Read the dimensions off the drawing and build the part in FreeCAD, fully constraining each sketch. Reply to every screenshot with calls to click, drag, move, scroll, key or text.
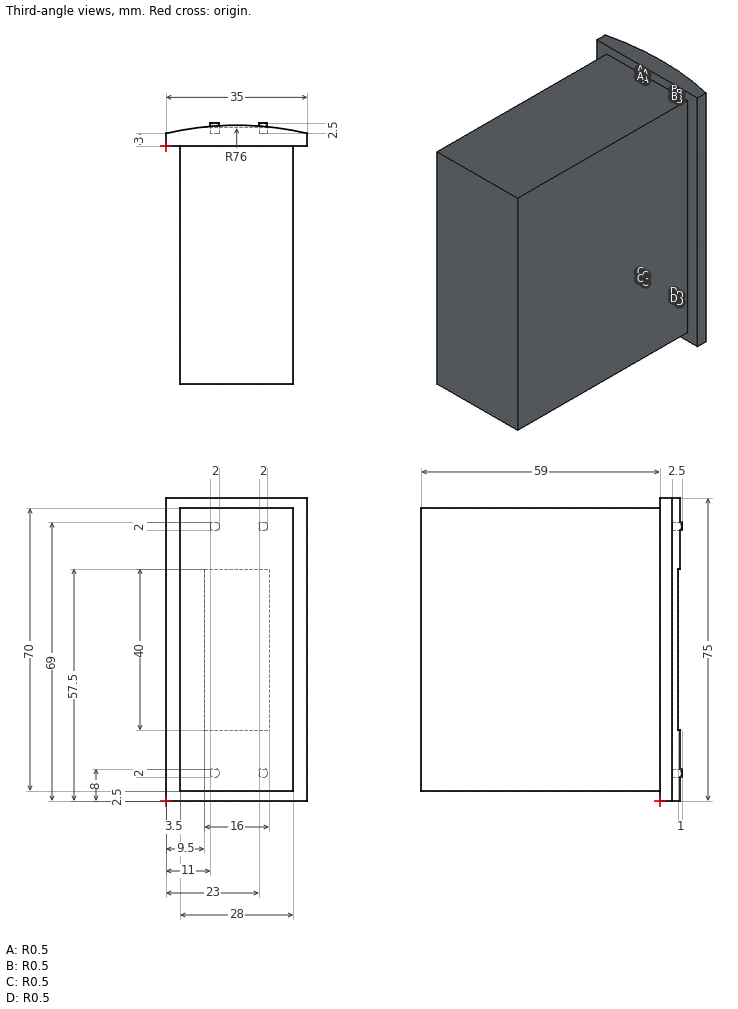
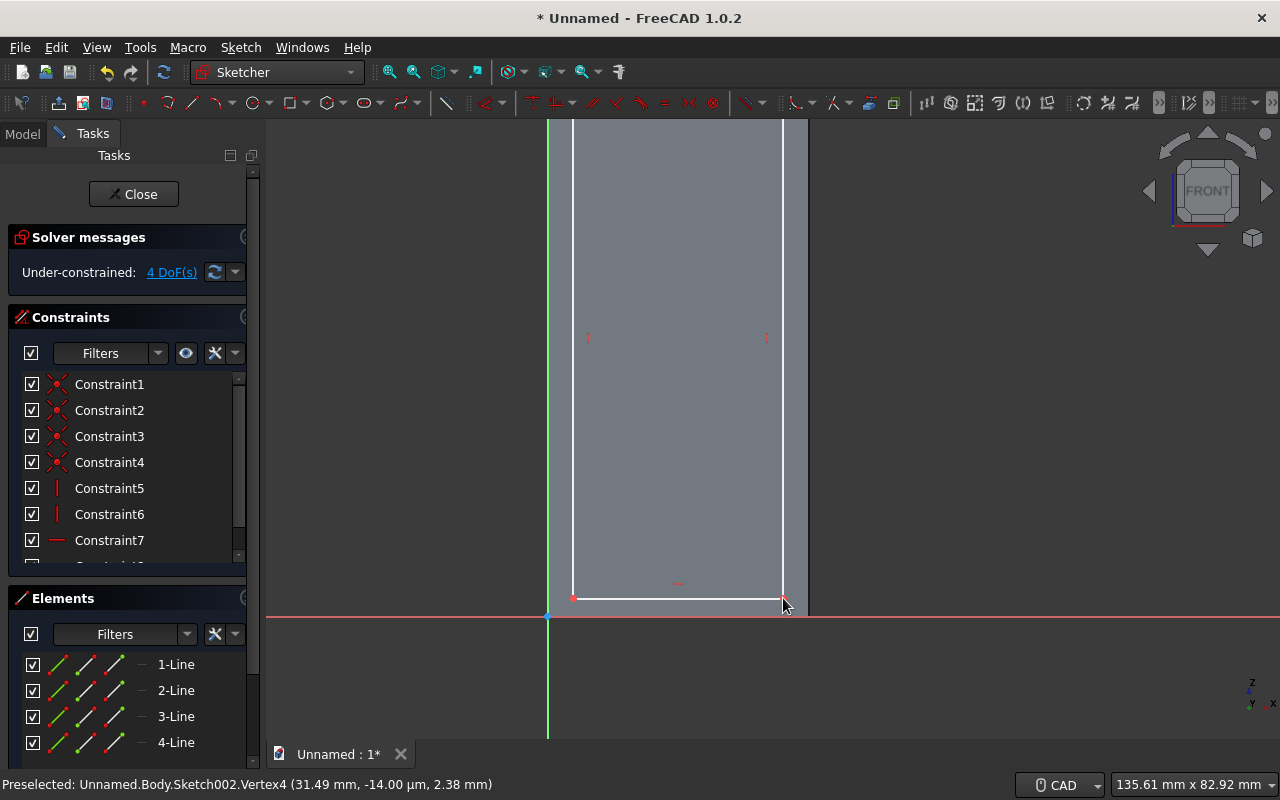
key(d)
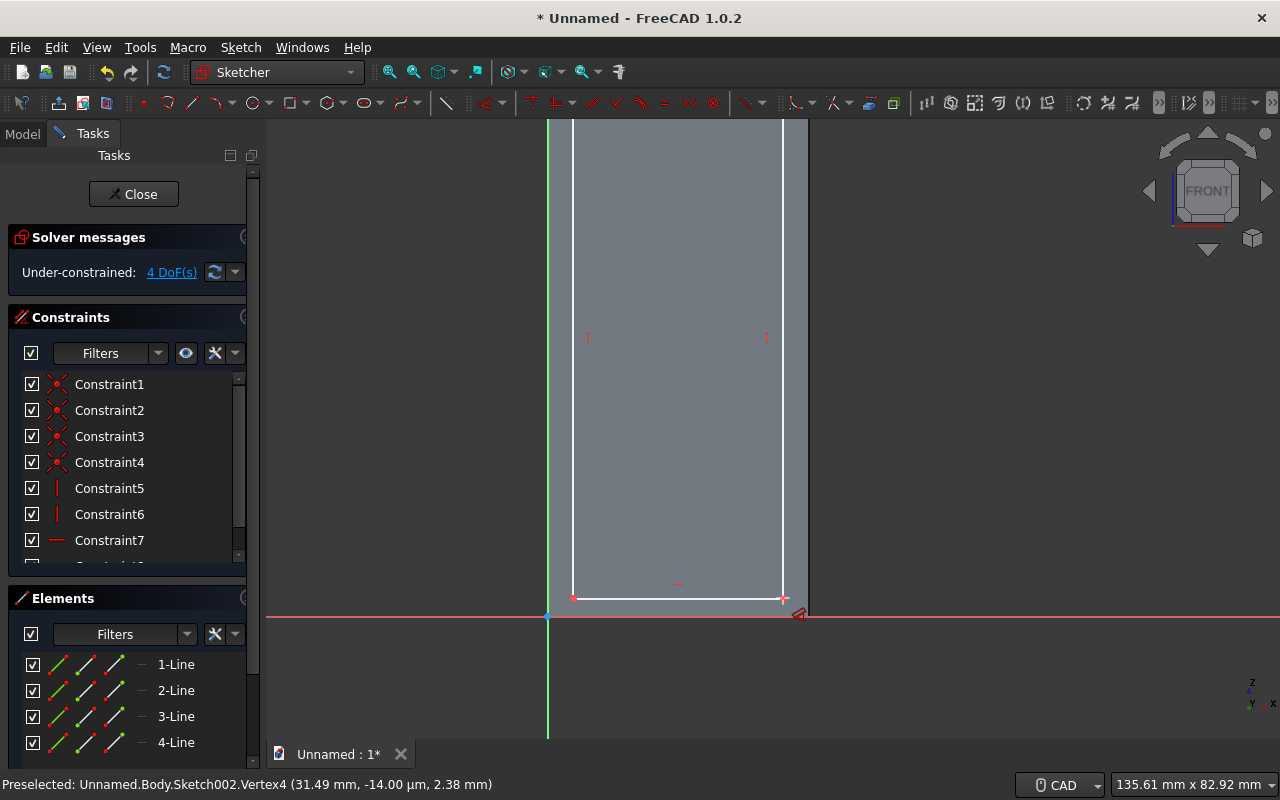
click(573, 233)
click(607, 373)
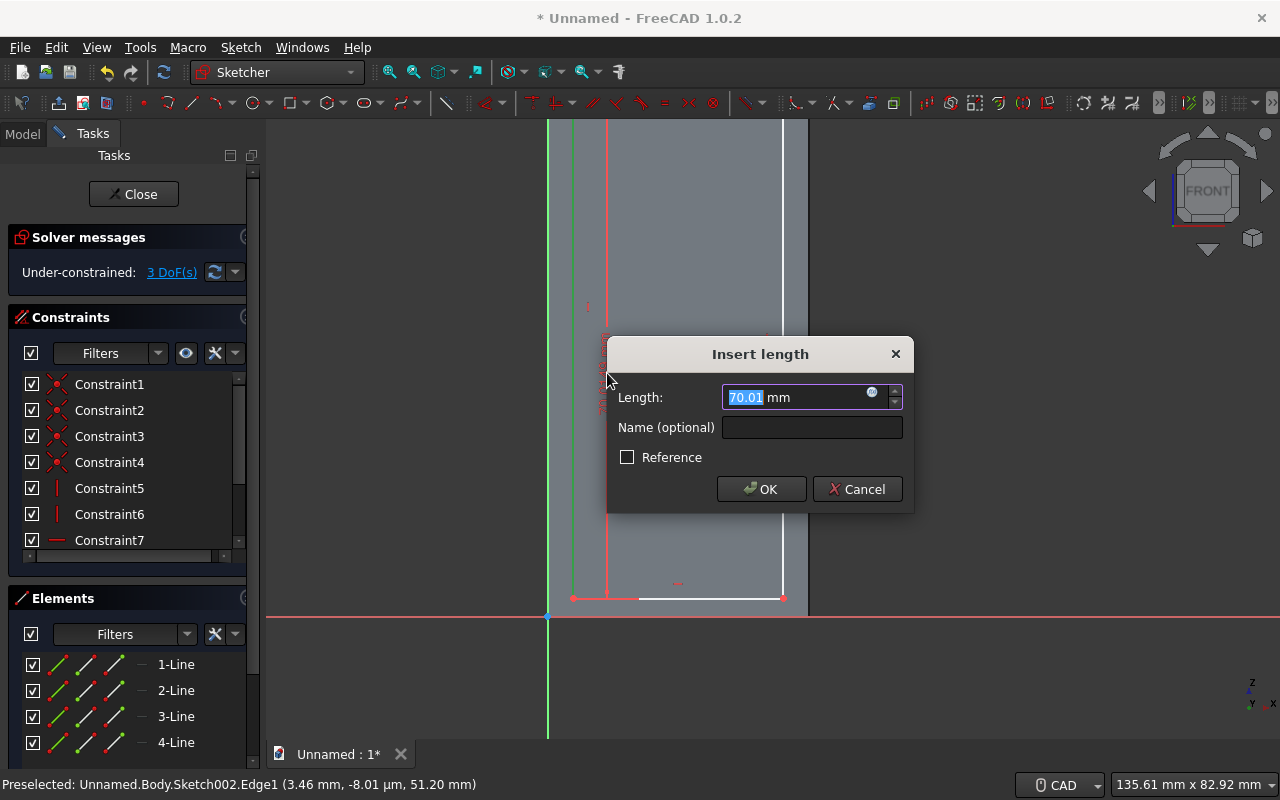
text(70)
key(Return)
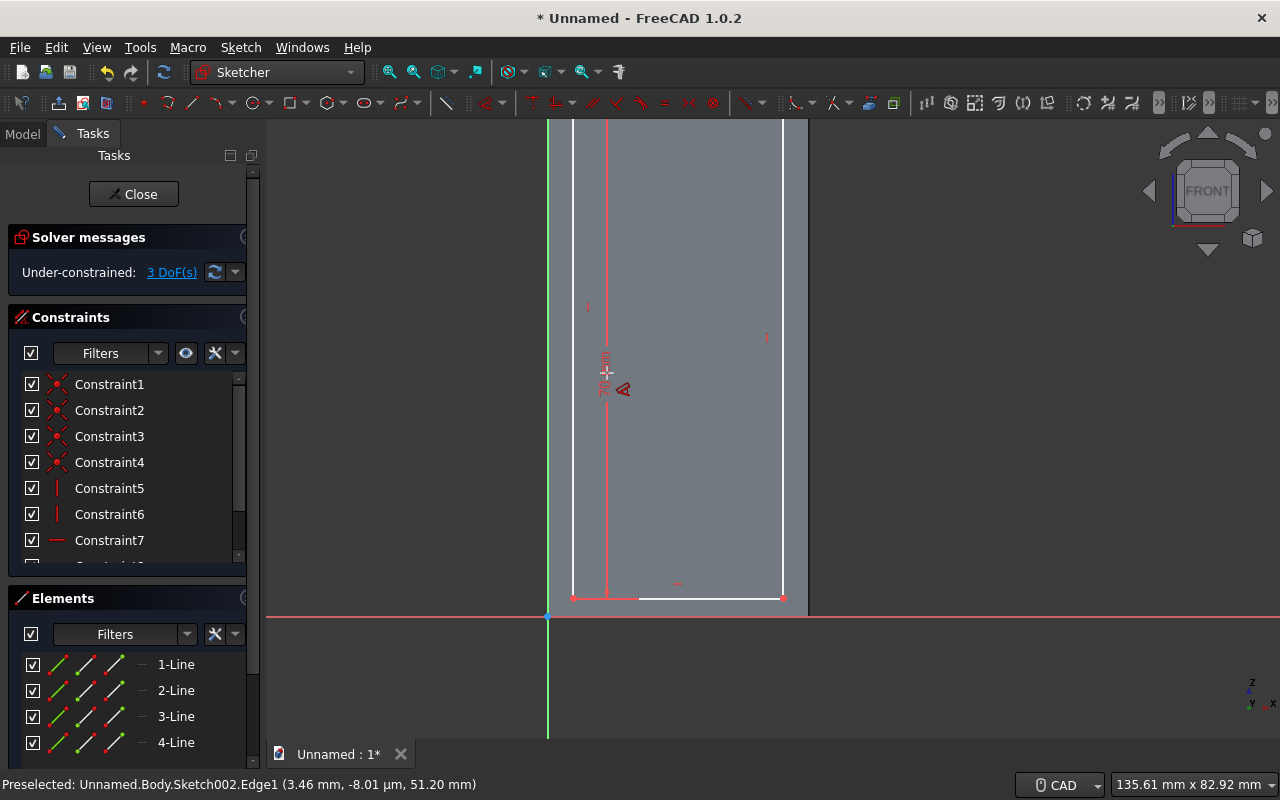
click(636, 599)
click(678, 633)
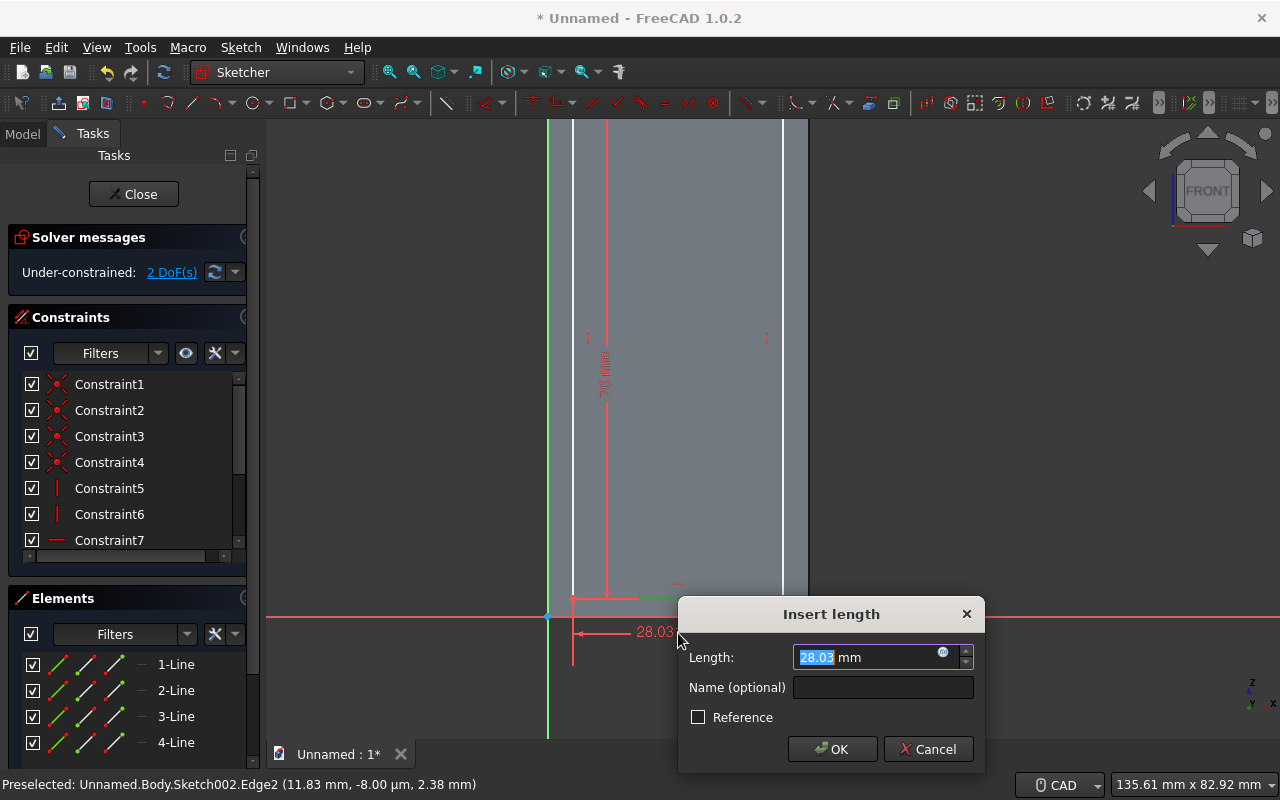
text(28)
key(Return)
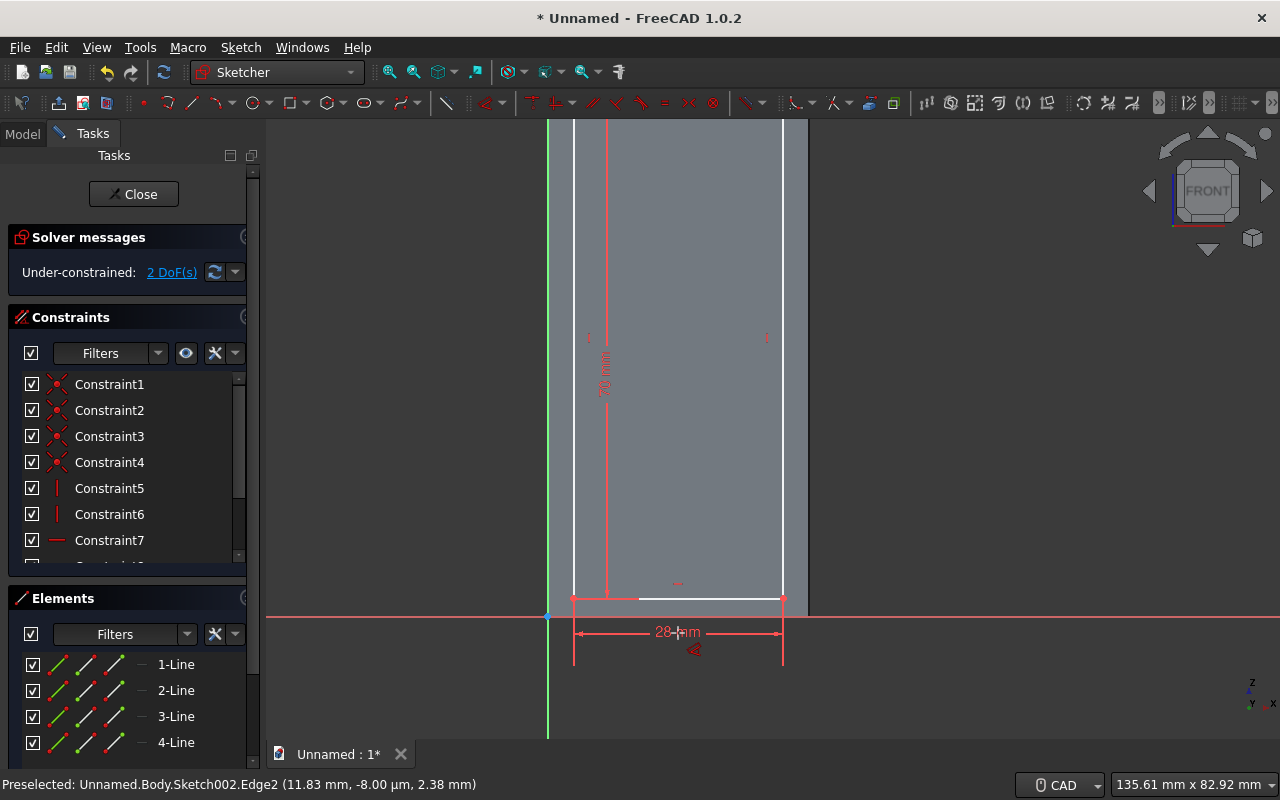
scroll(784, 598, down, 2)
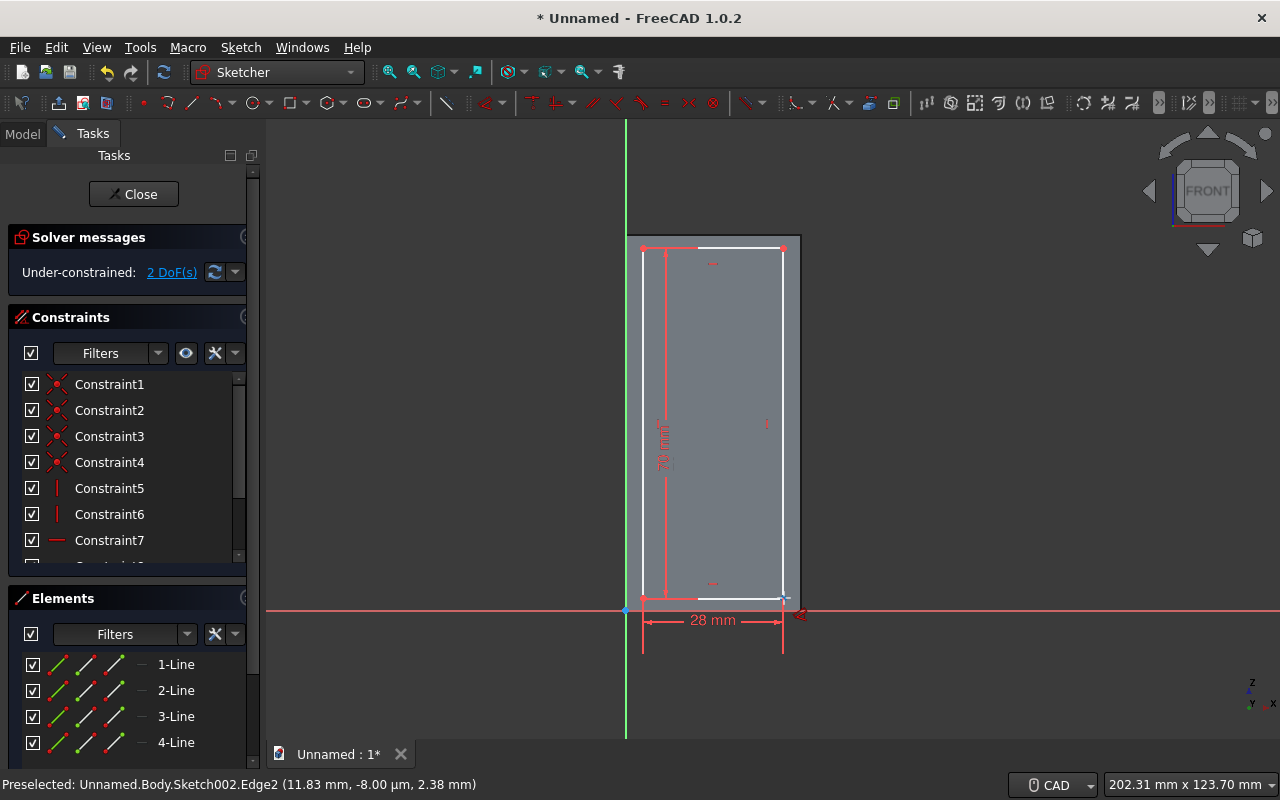
scroll(643, 248, up, 5)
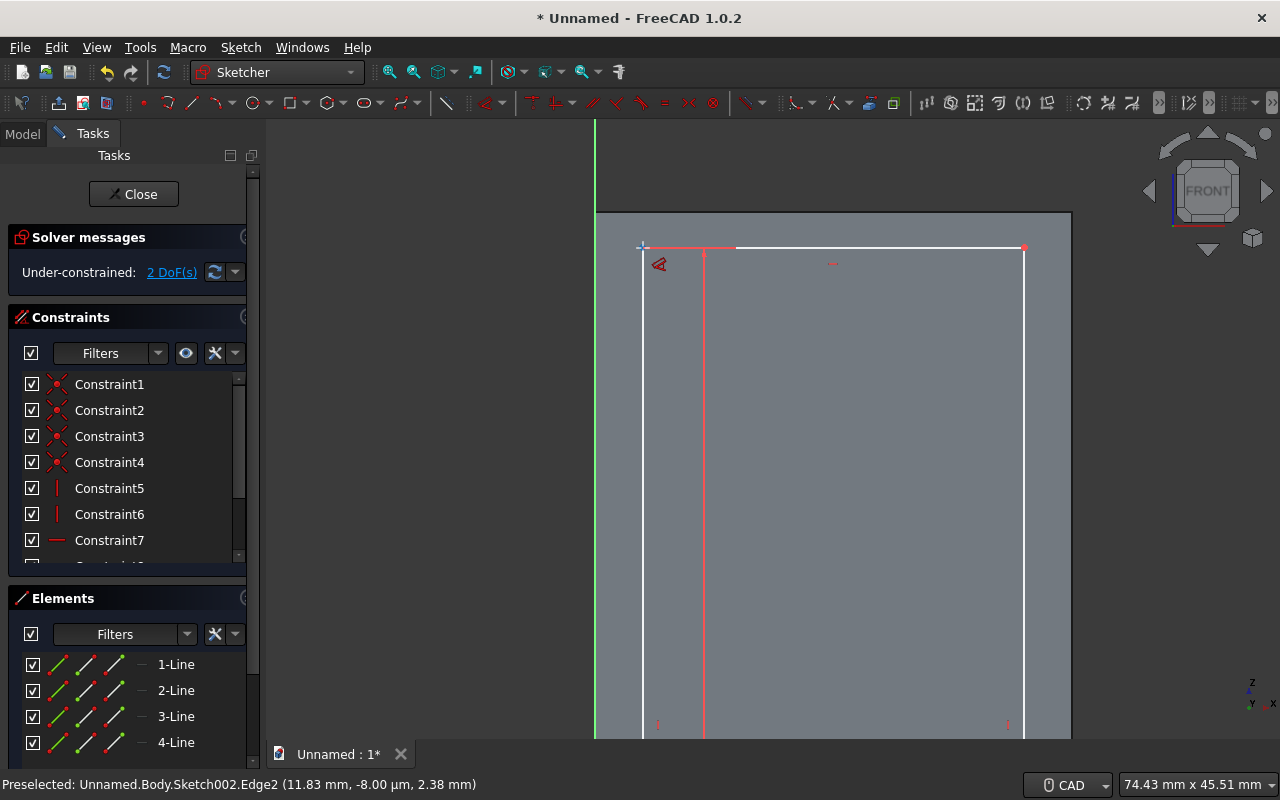
click(643, 248)
click(619, 214)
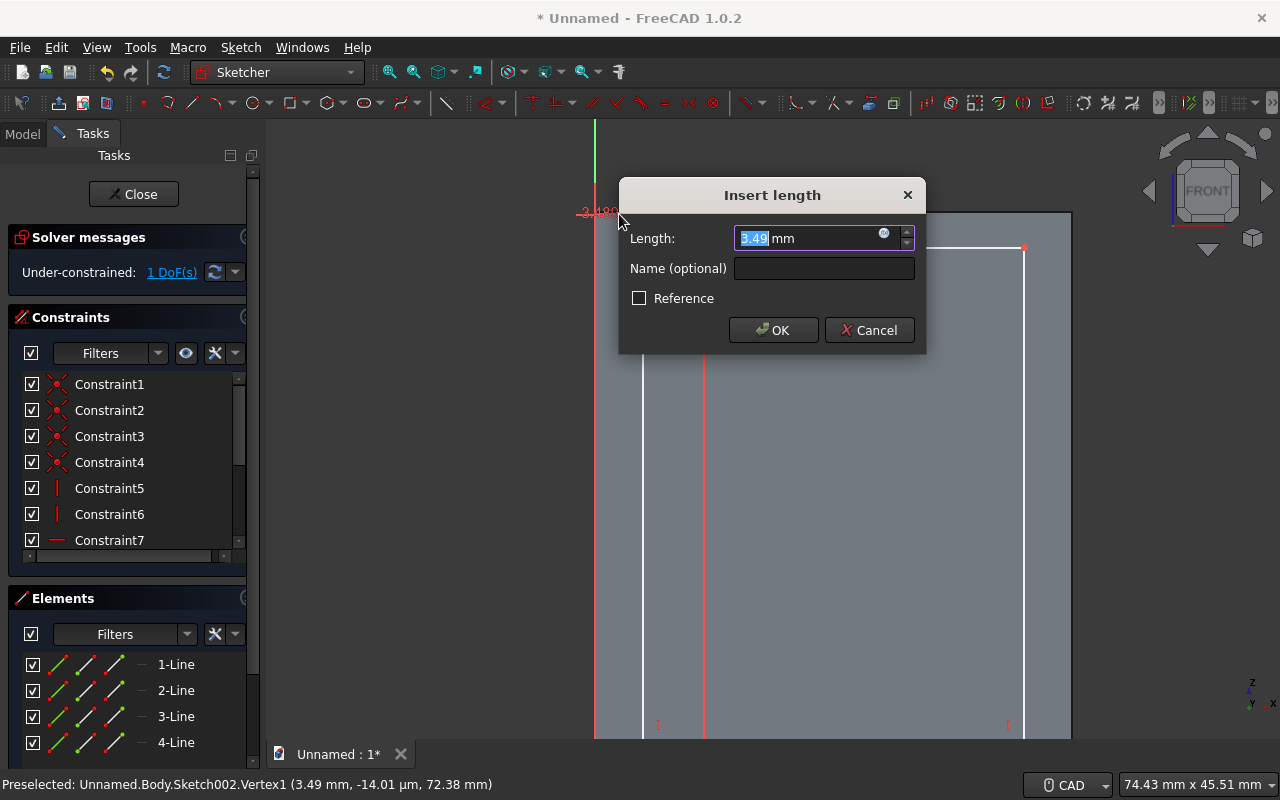
text(3.5)
key(Return)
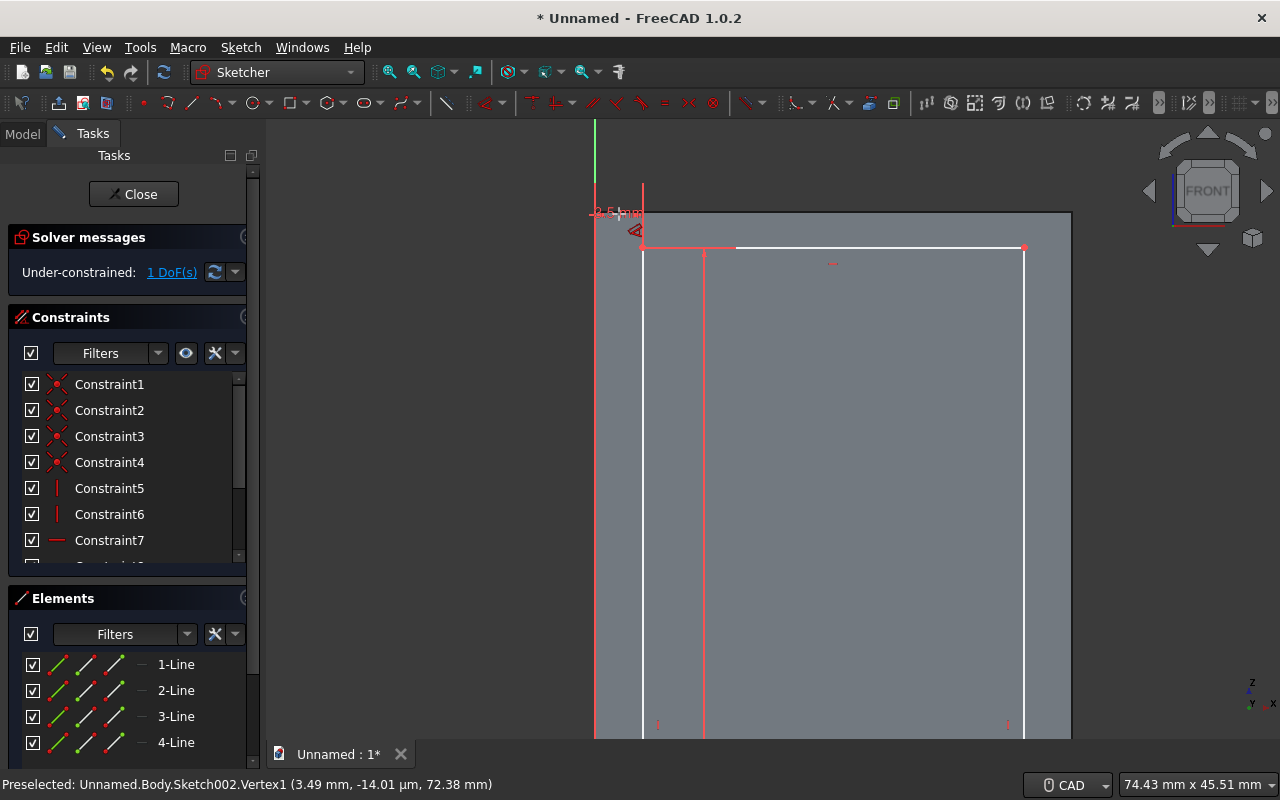
scroll(643, 248, down, 5)